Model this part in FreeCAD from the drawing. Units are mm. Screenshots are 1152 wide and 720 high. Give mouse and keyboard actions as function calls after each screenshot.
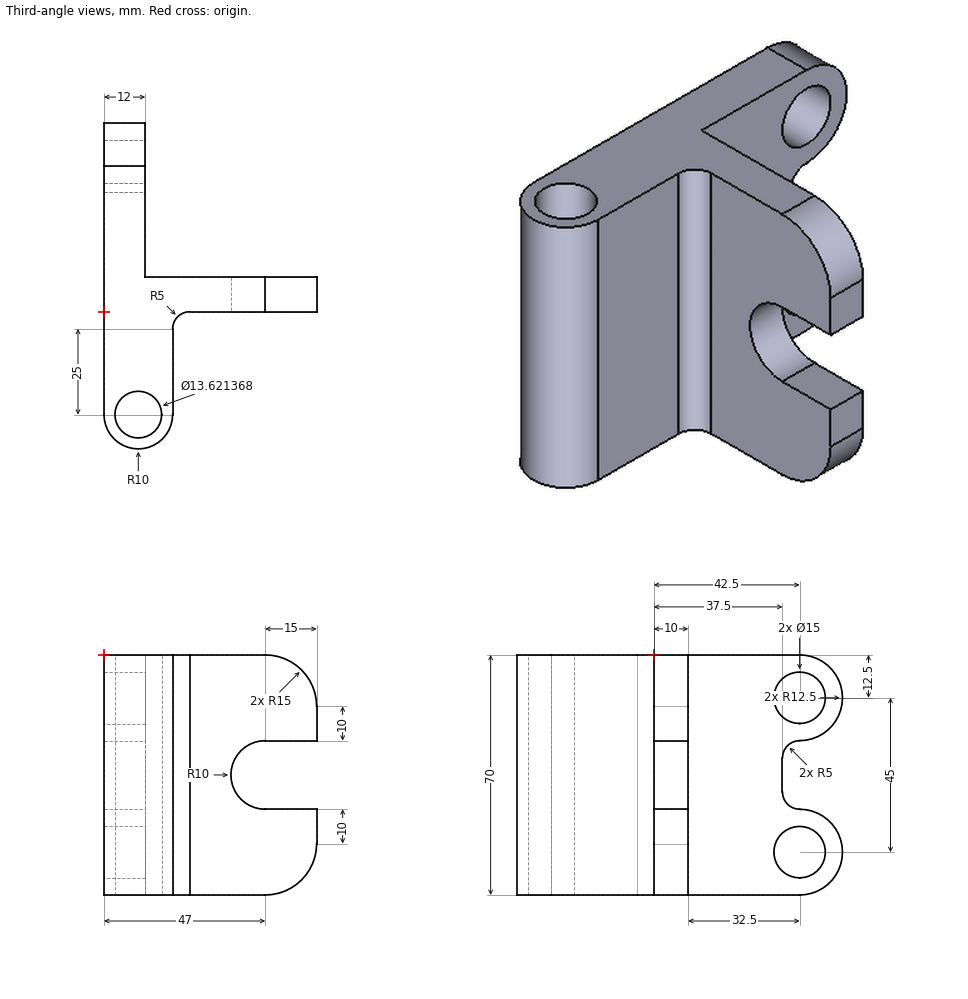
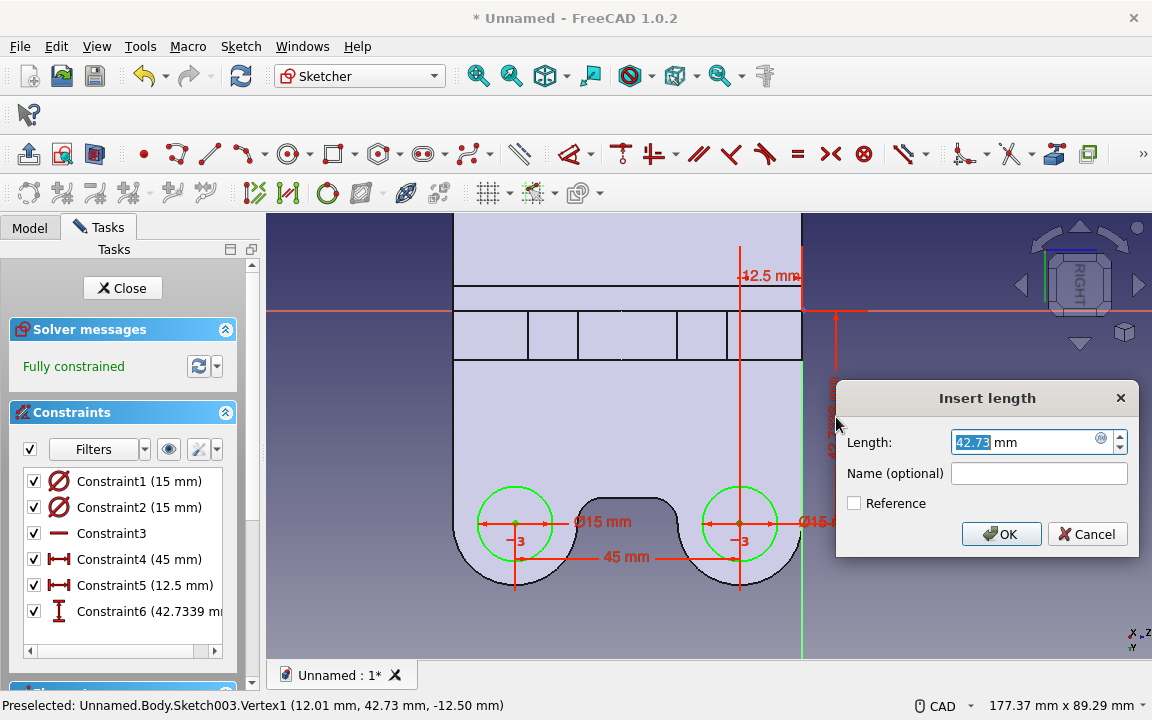
text(42.5)
key(Return)
key(Escape)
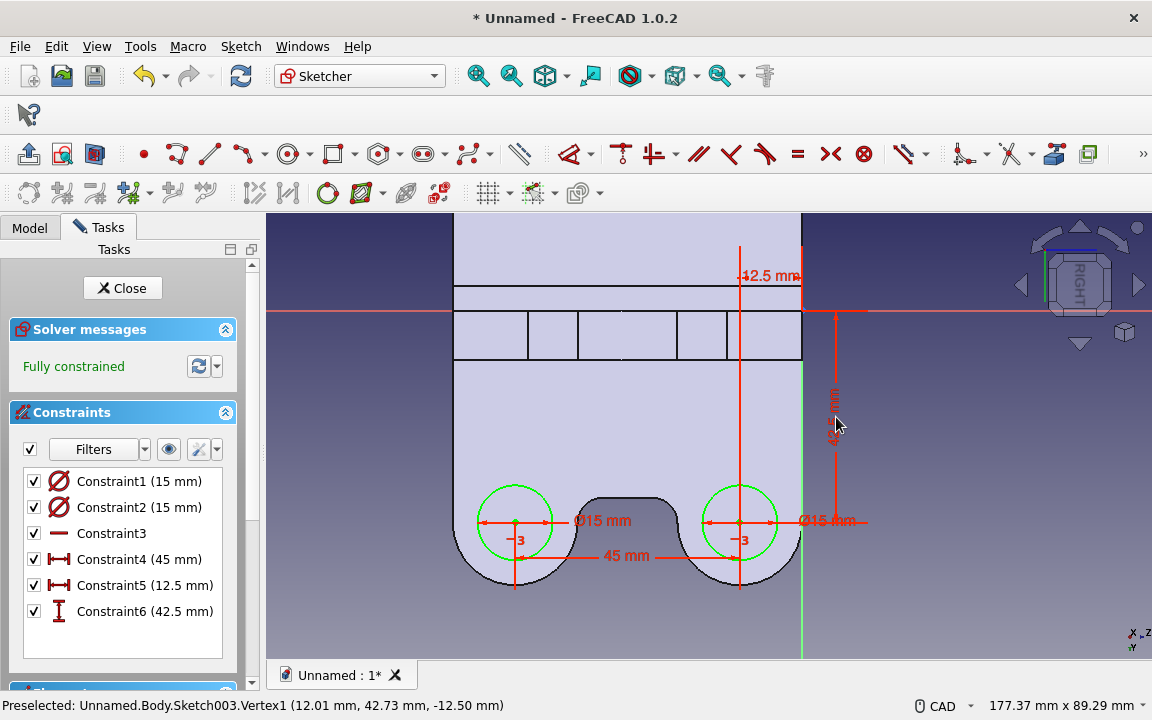
click(123, 288)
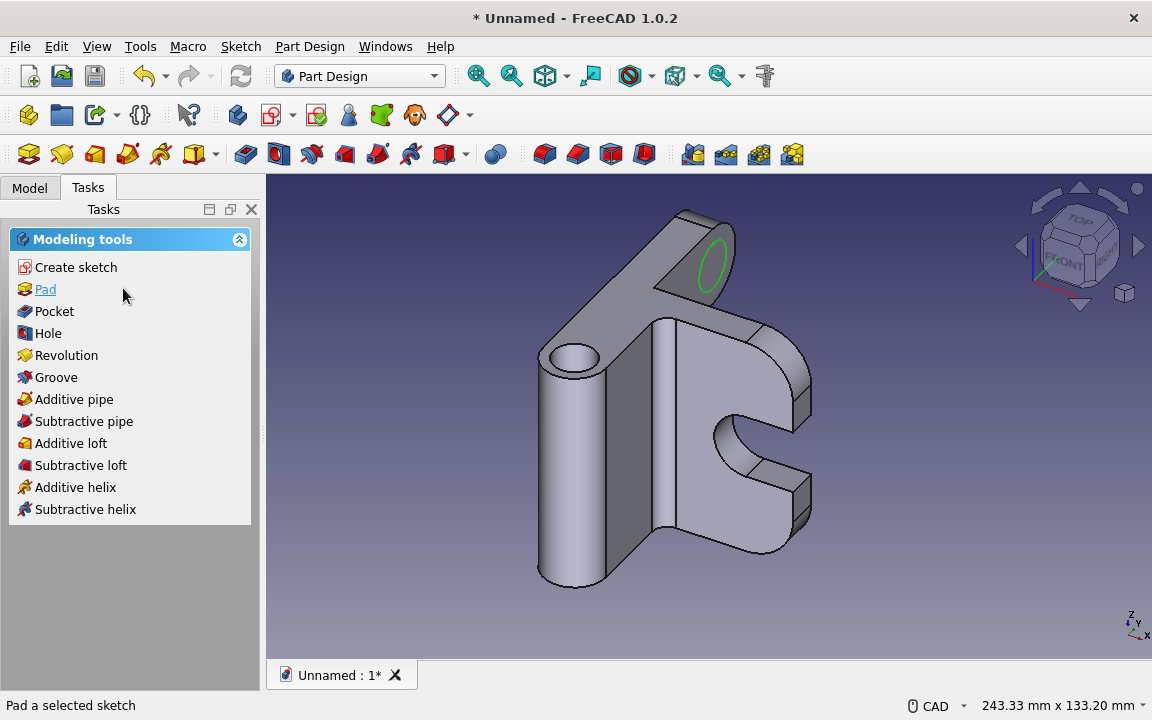
click(246, 154)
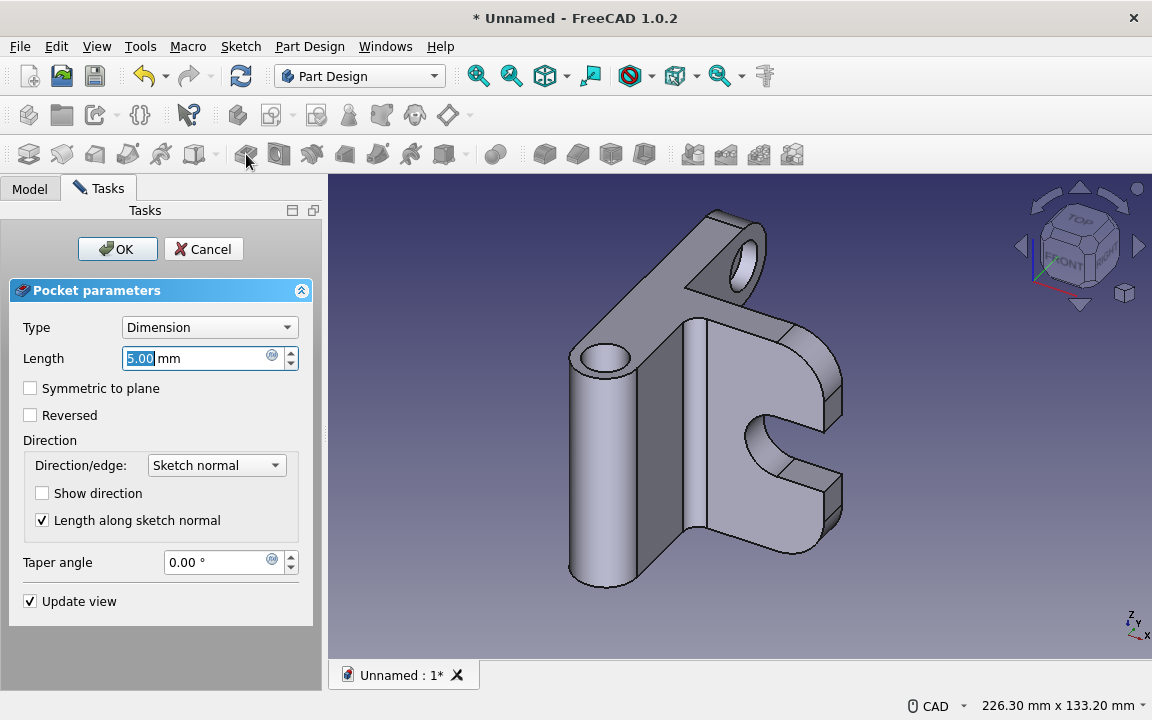
text(12)
key(Tab)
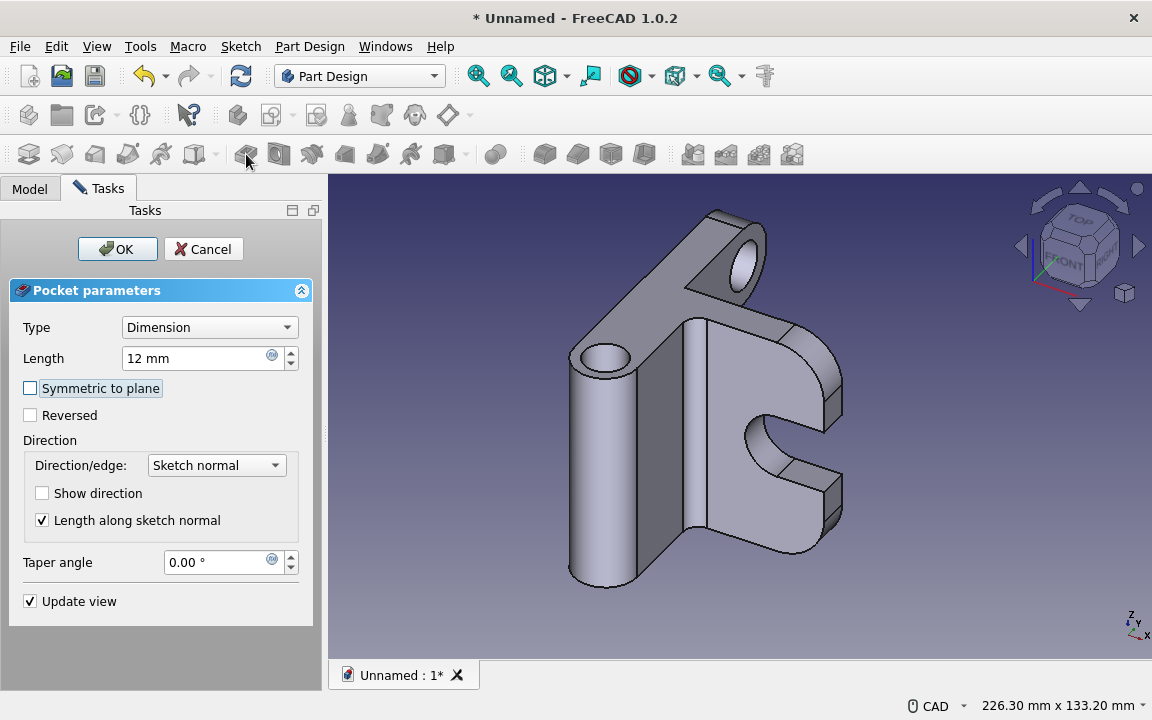
click(118, 249)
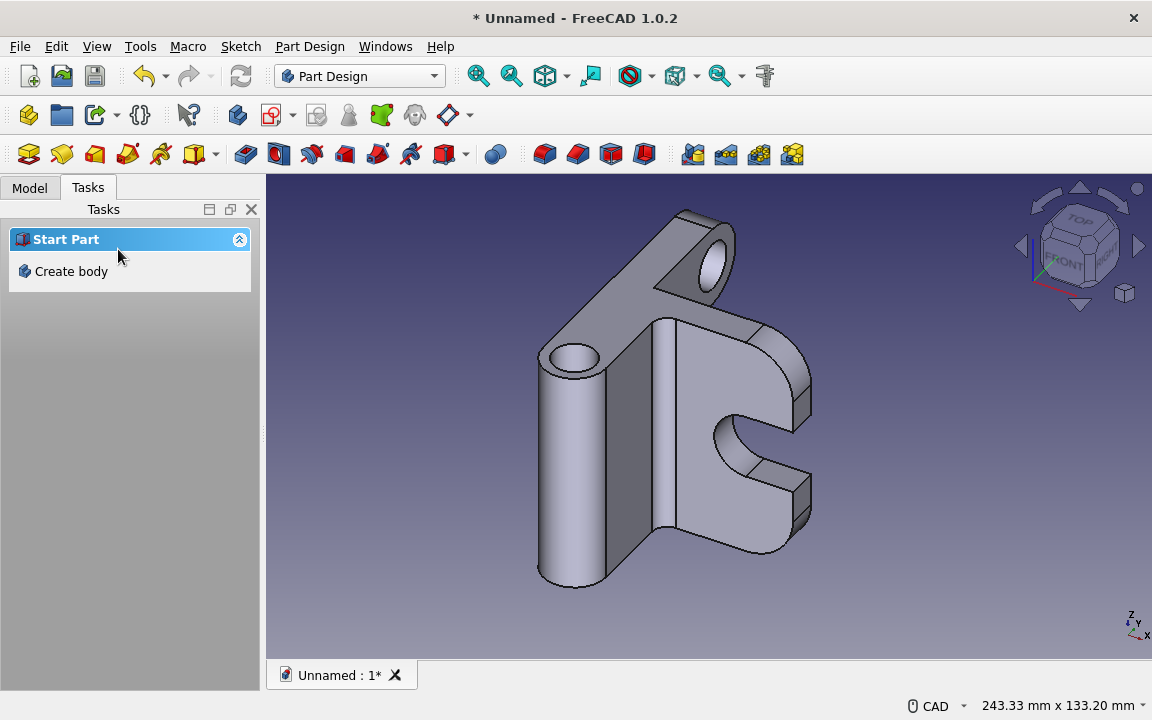
key(0)